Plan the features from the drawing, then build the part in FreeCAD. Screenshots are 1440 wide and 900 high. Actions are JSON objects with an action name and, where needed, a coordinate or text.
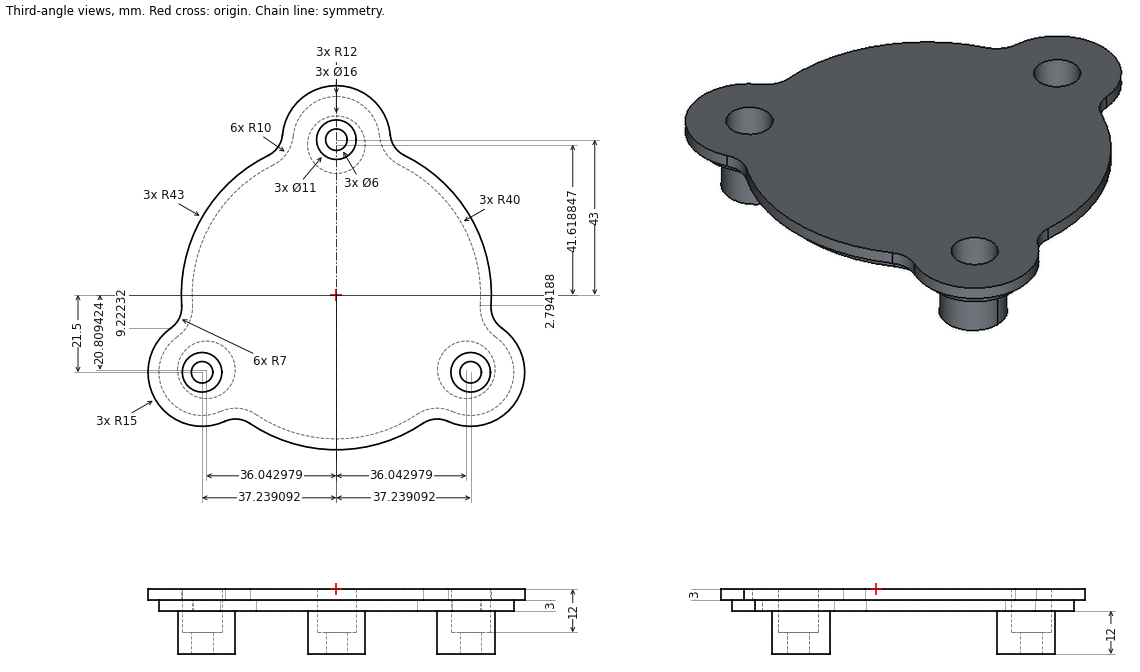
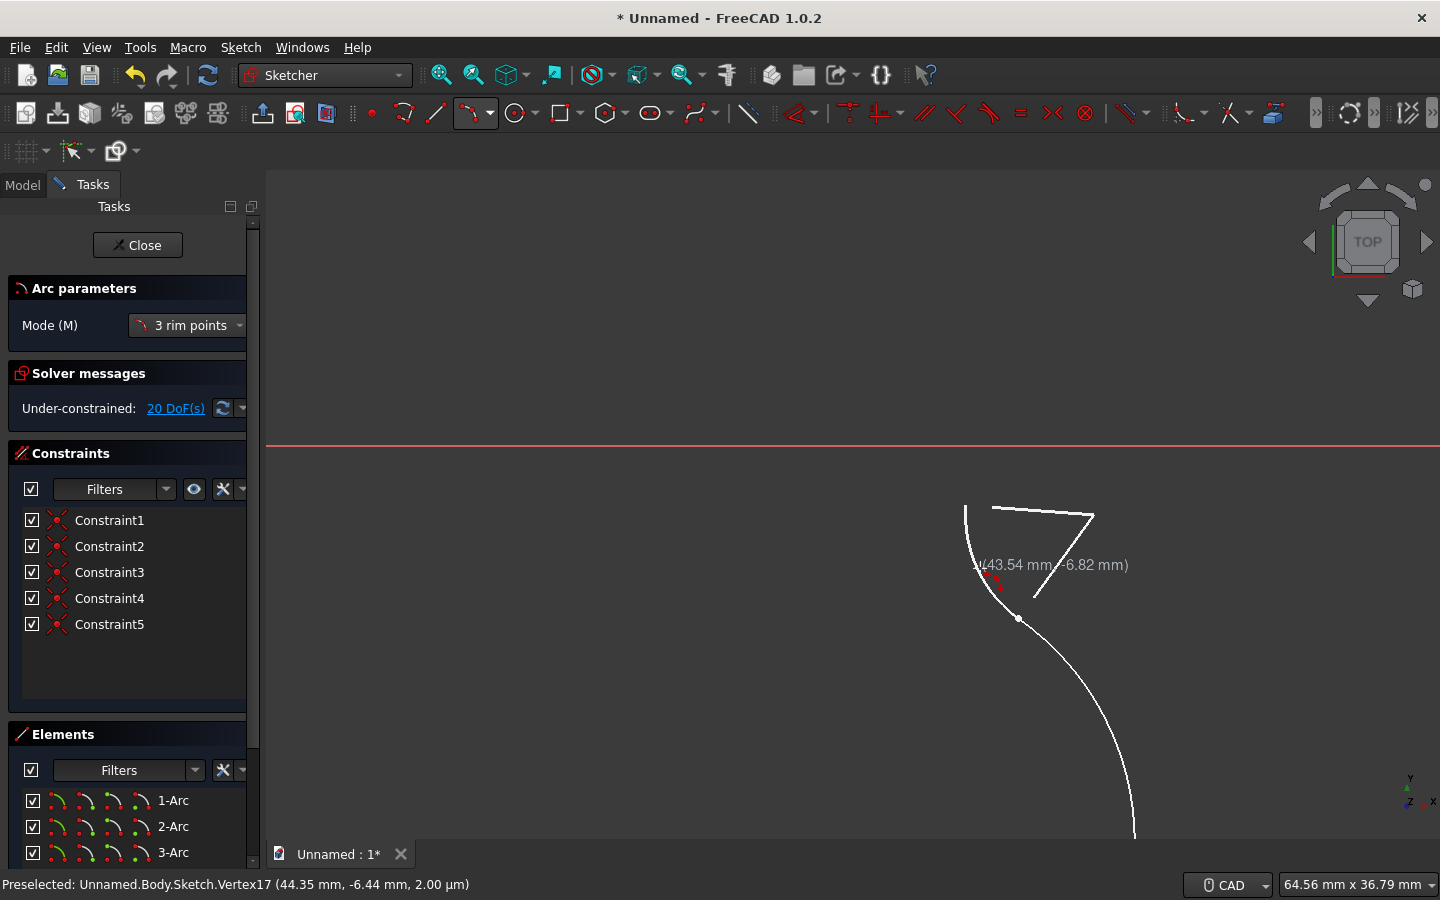
{"action": "left_click", "coordinate": [978, 564]}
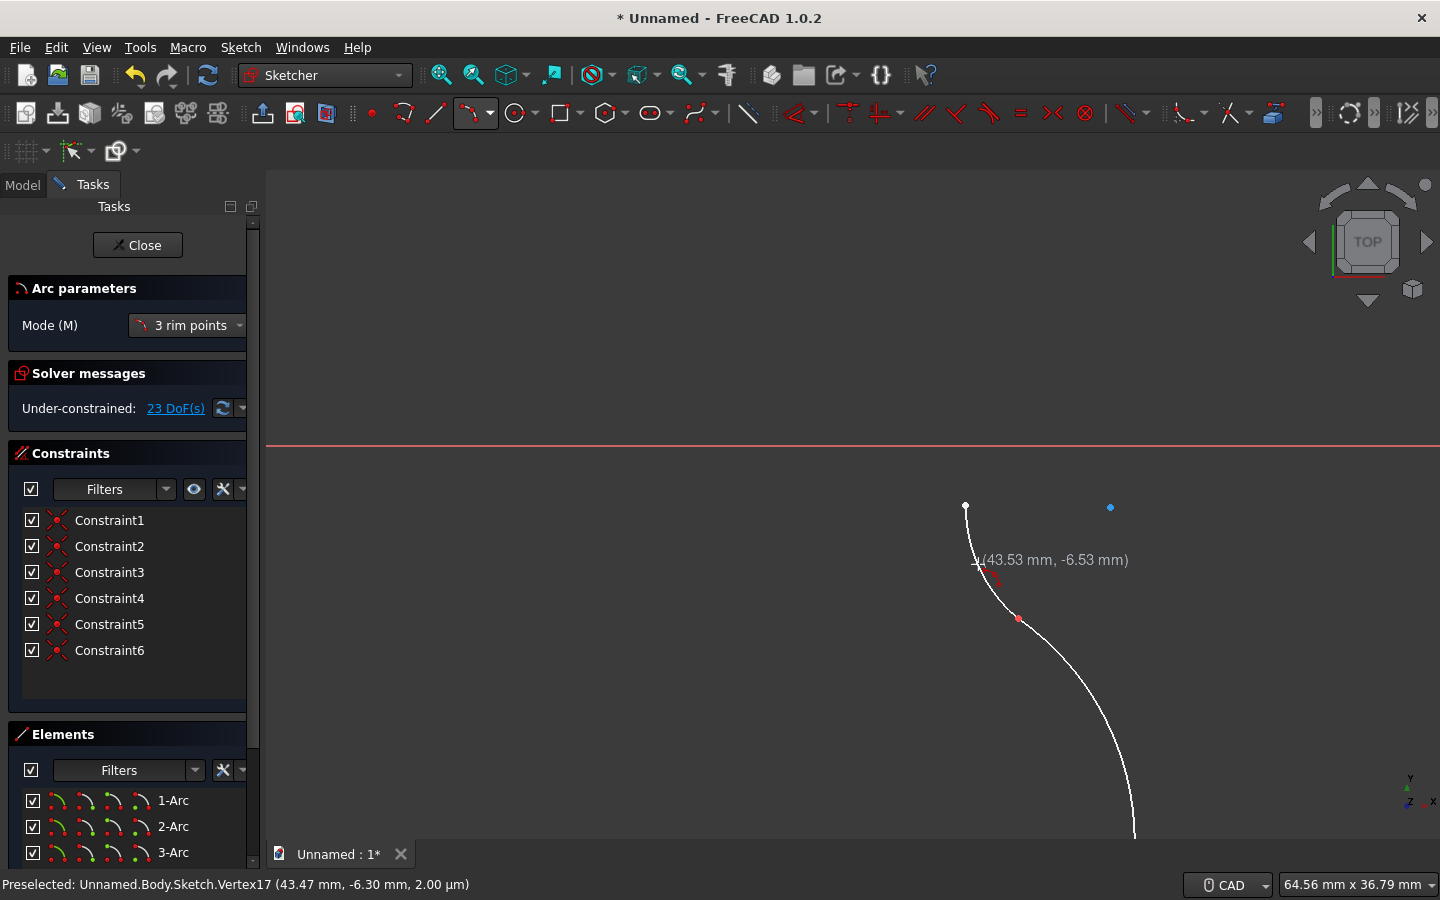
{"action": "scroll", "coordinate": [980, 568], "scroll_direction": "down", "scroll_amount": 7}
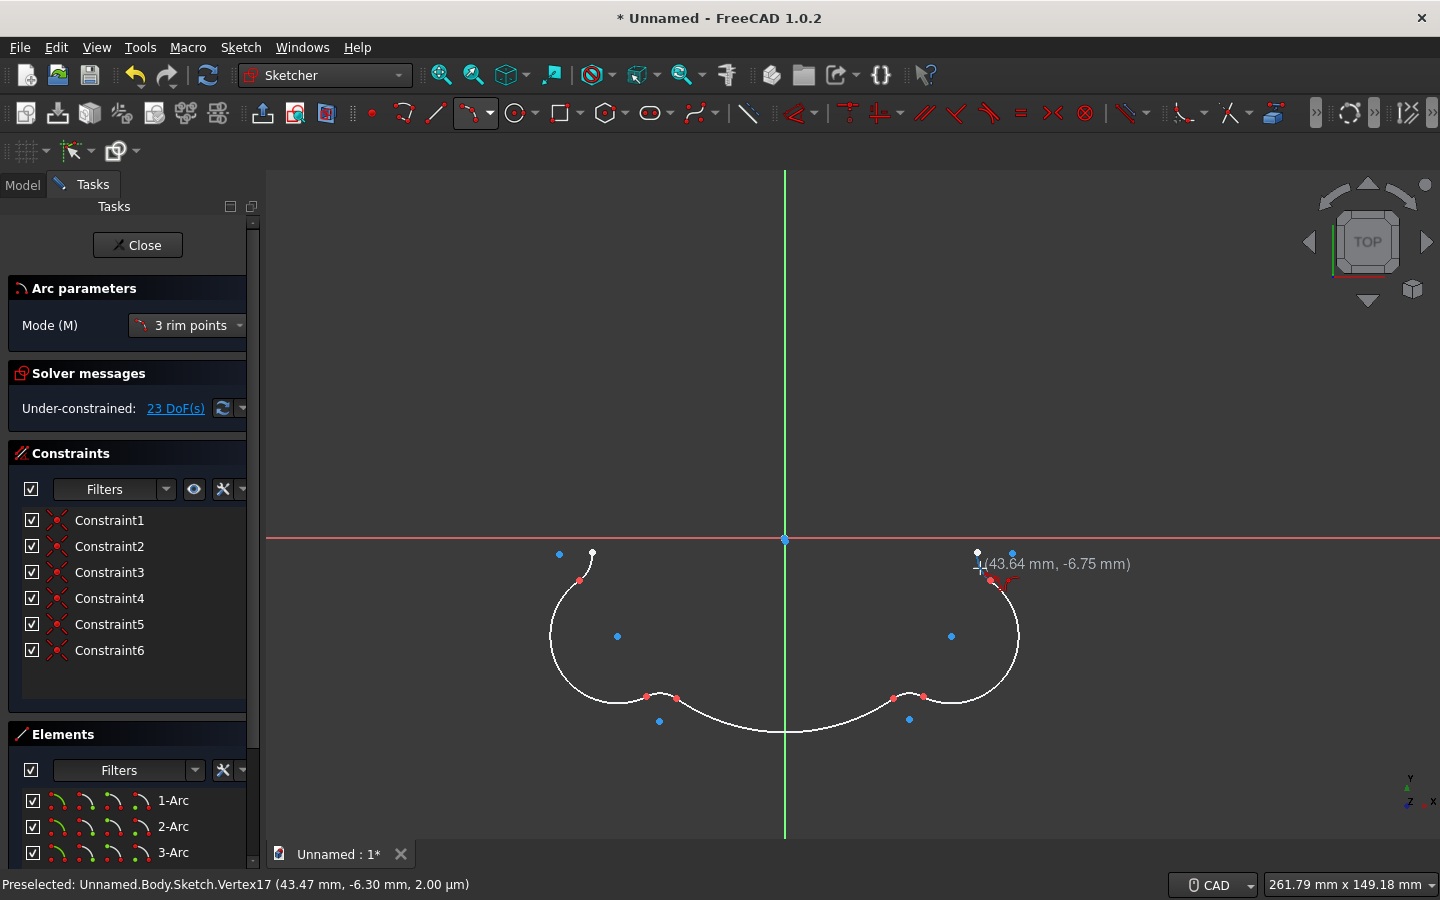
{"action": "left_click", "coordinate": [977, 553]}
{"action": "left_click", "coordinate": [869, 365]}
{"action": "left_click", "coordinate": [952, 442]}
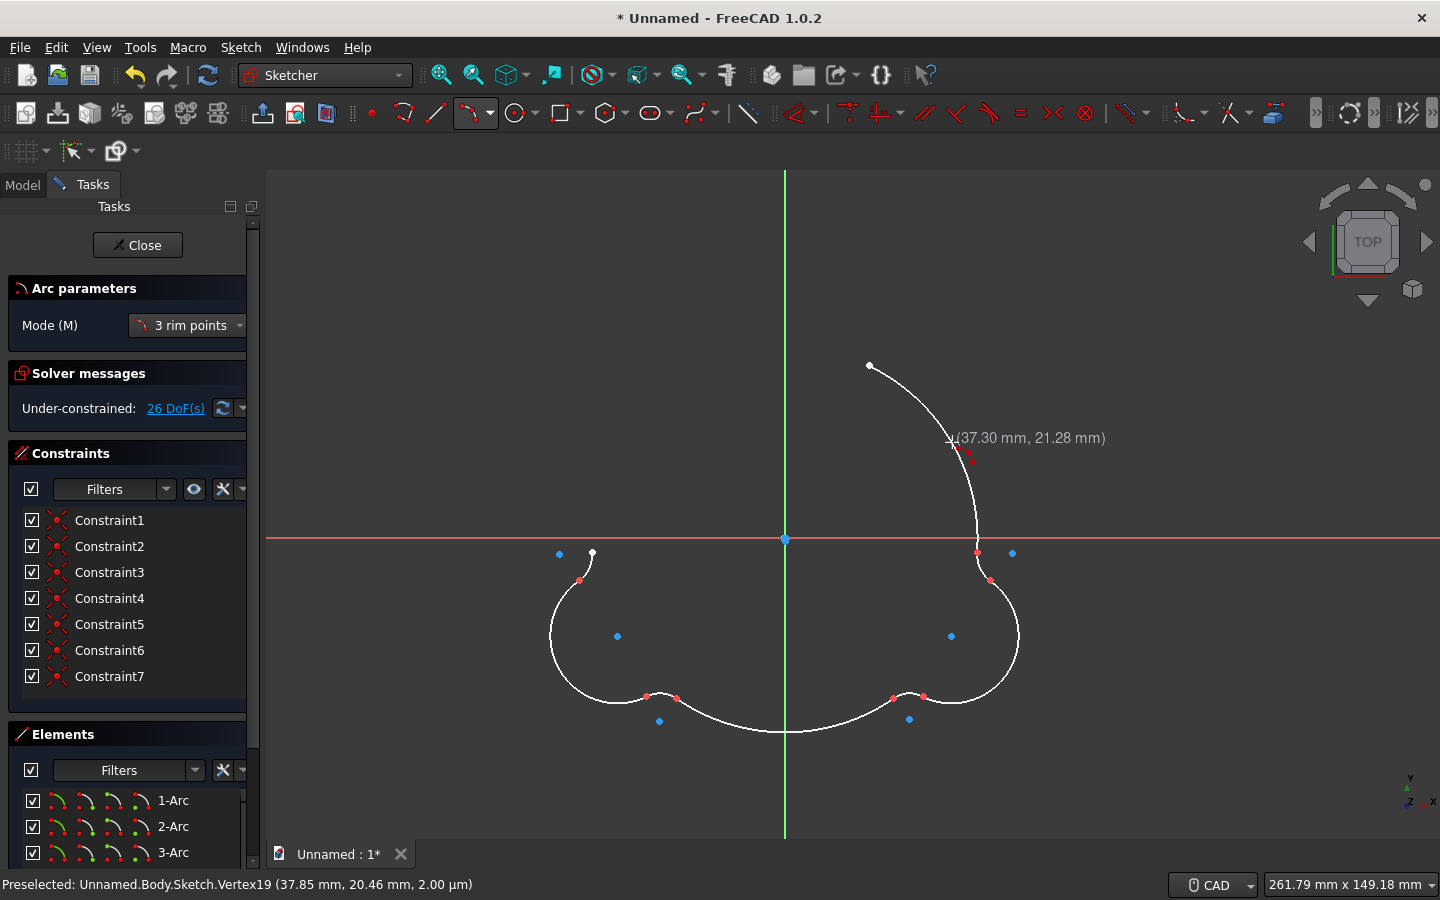
{"action": "left_click", "coordinate": [869, 366]}
{"action": "left_click", "coordinate": [852, 340]}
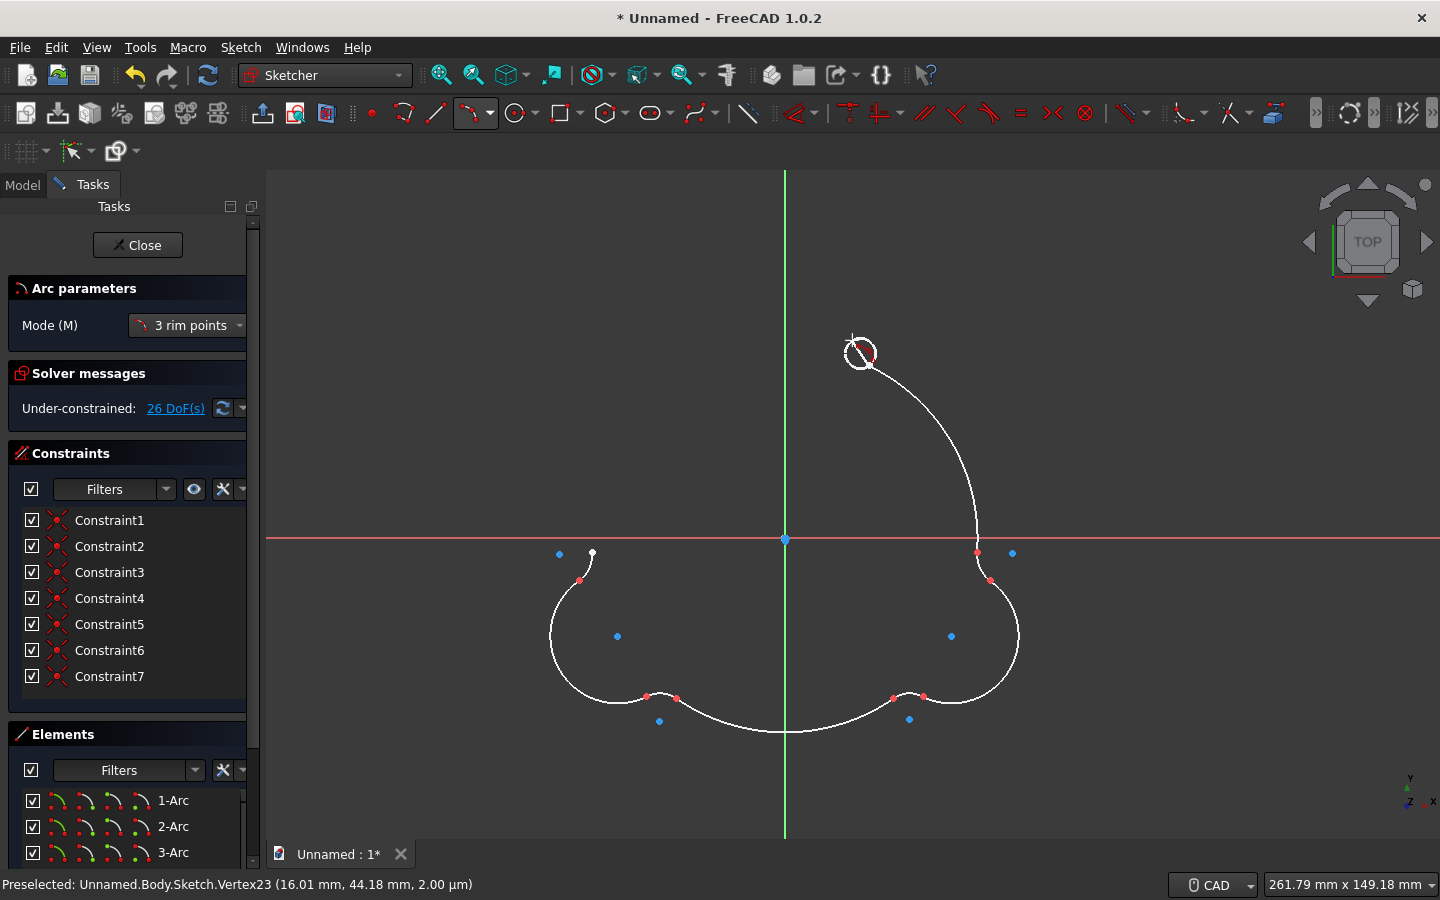
{"action": "scroll", "coordinate": [857, 355], "scroll_direction": "up", "scroll_amount": 7}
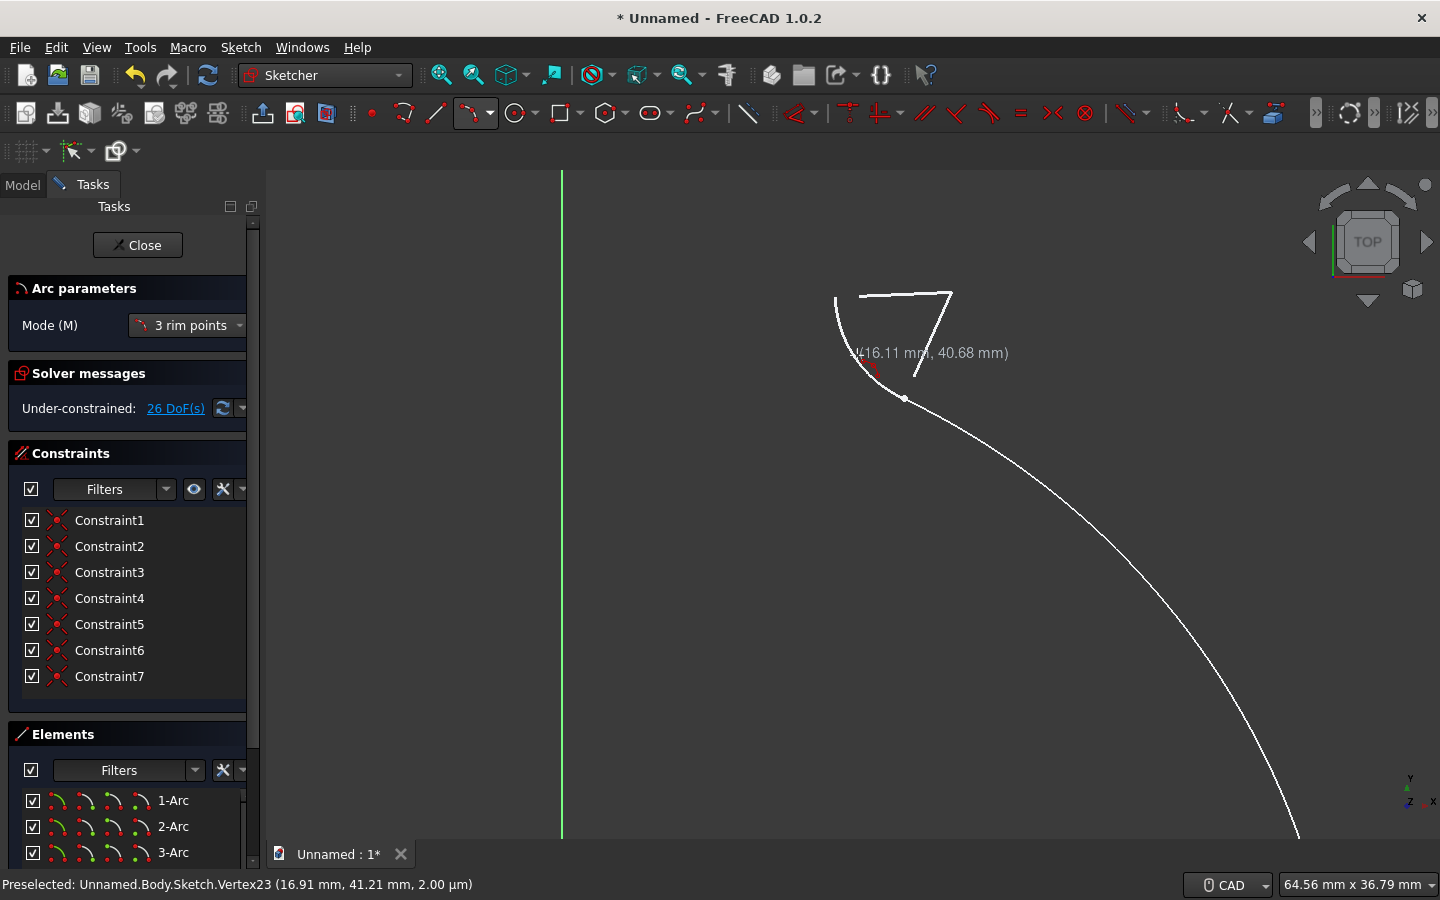
{"action": "left_click", "coordinate": [856, 353]}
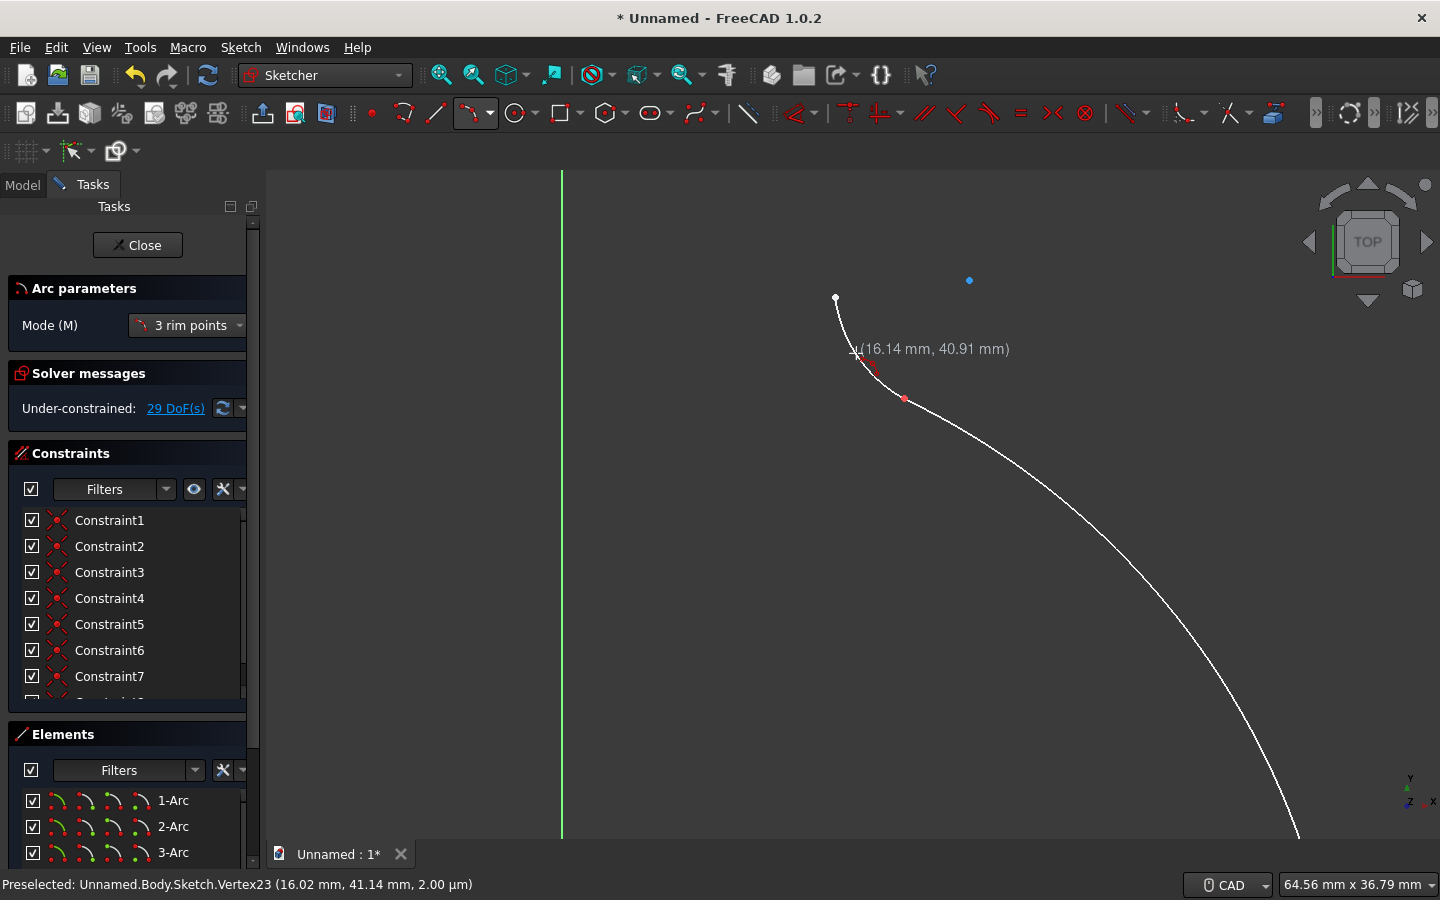
{"action": "scroll", "coordinate": [857, 355], "scroll_direction": "down", "scroll_amount": 7}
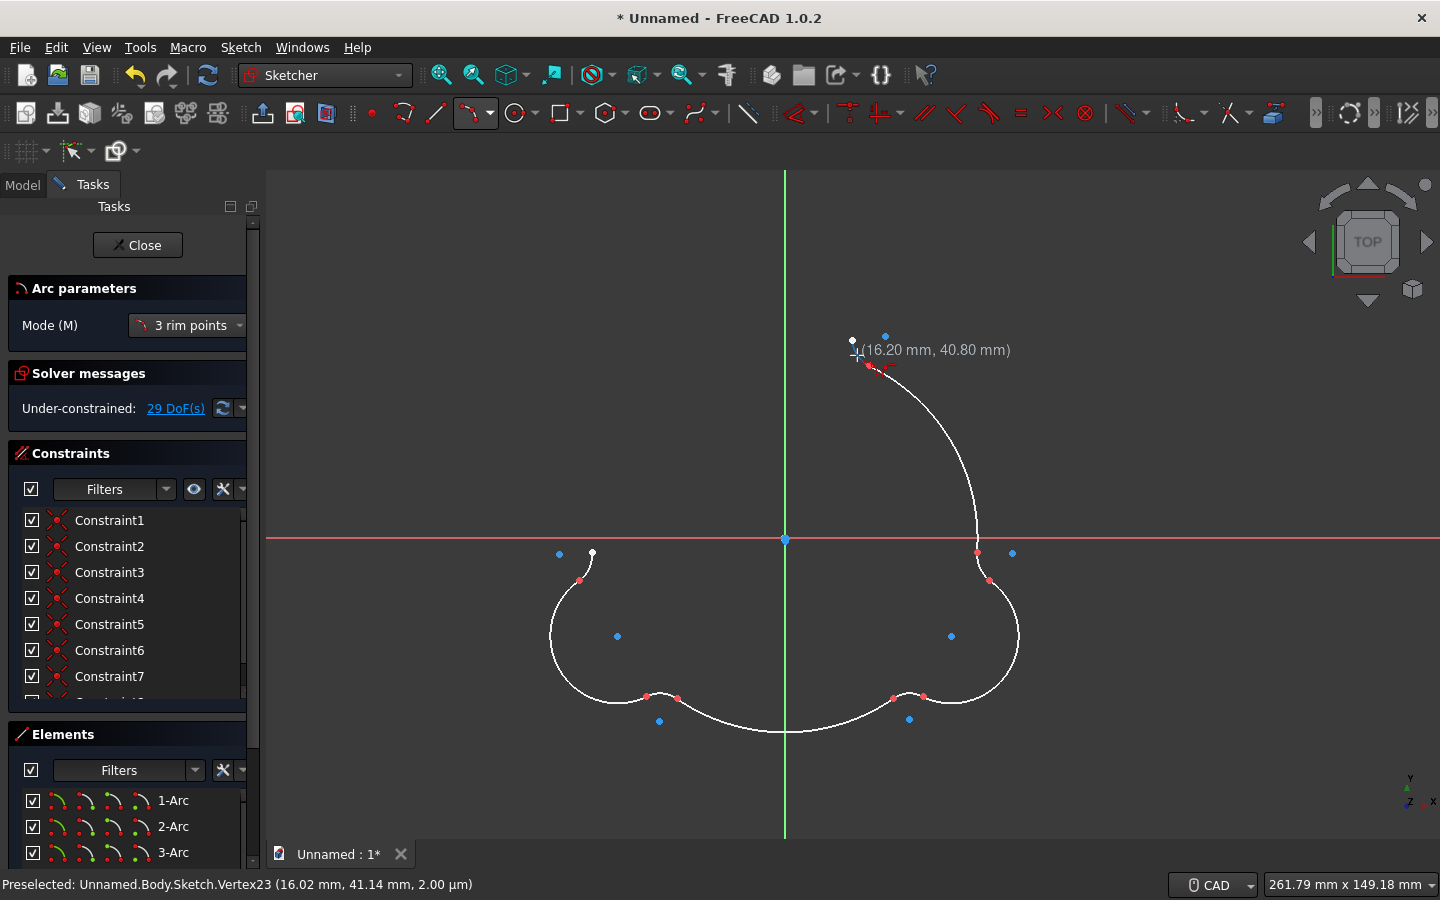
{"action": "left_click", "coordinate": [852, 341]}
{"action": "left_click", "coordinate": [718, 340]}
{"action": "left_click", "coordinate": [804, 281]}